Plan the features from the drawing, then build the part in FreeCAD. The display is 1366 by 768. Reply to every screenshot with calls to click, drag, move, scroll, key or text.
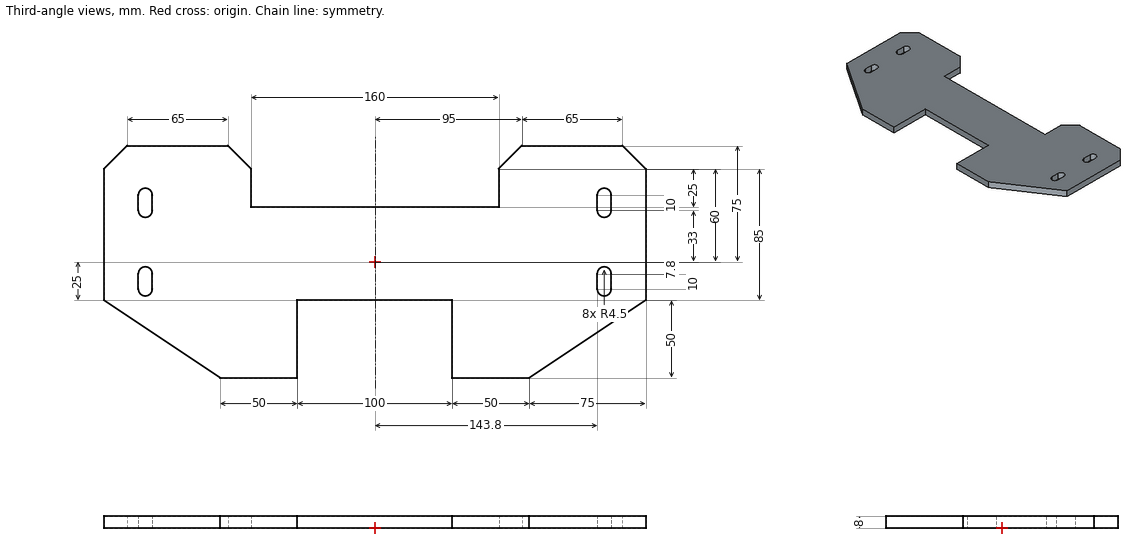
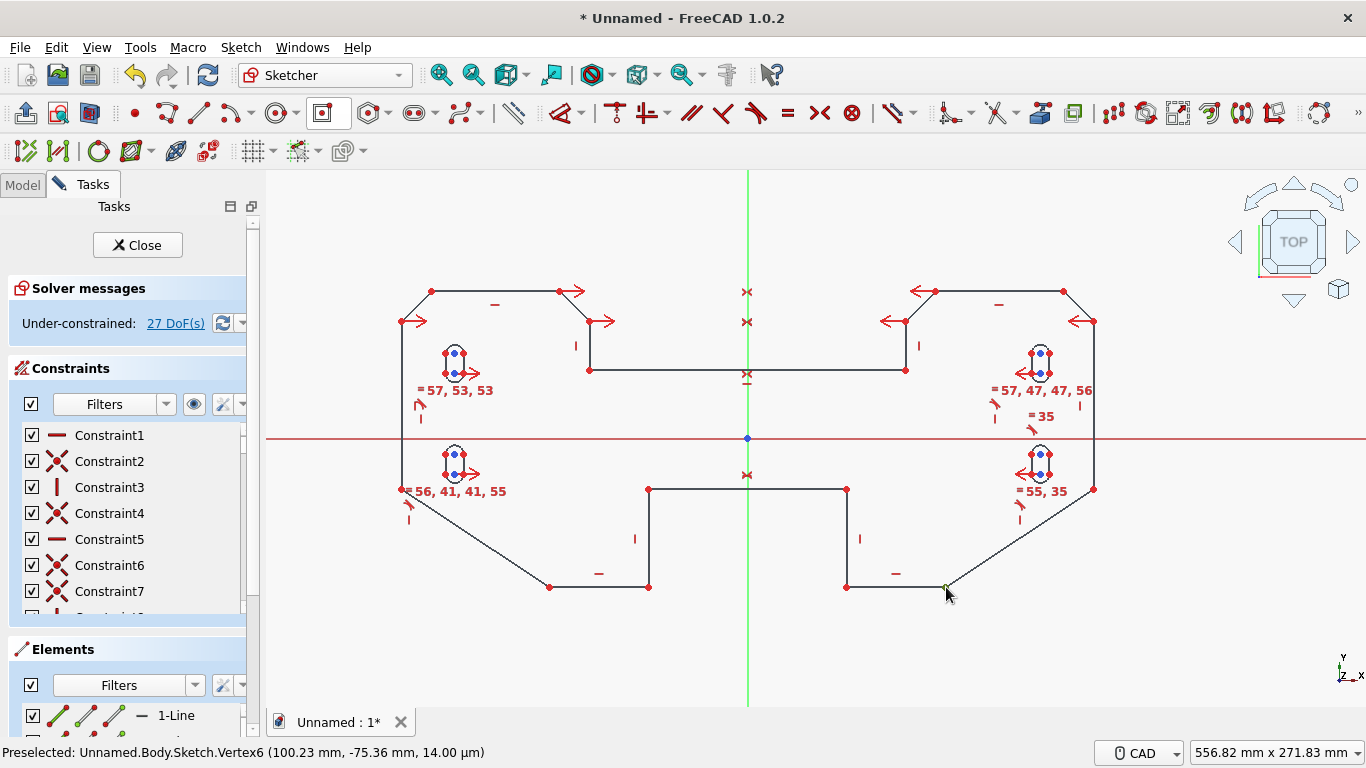
click(550, 587)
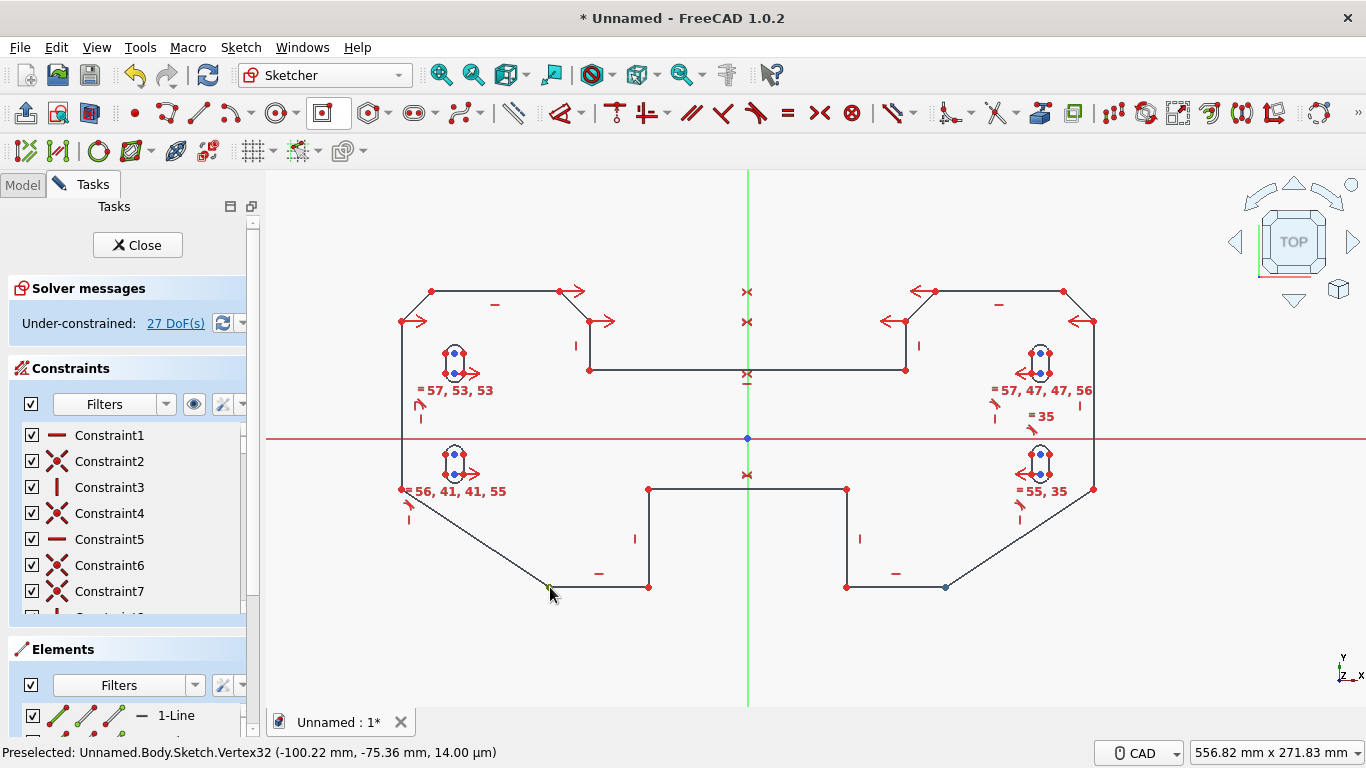
click(748, 645)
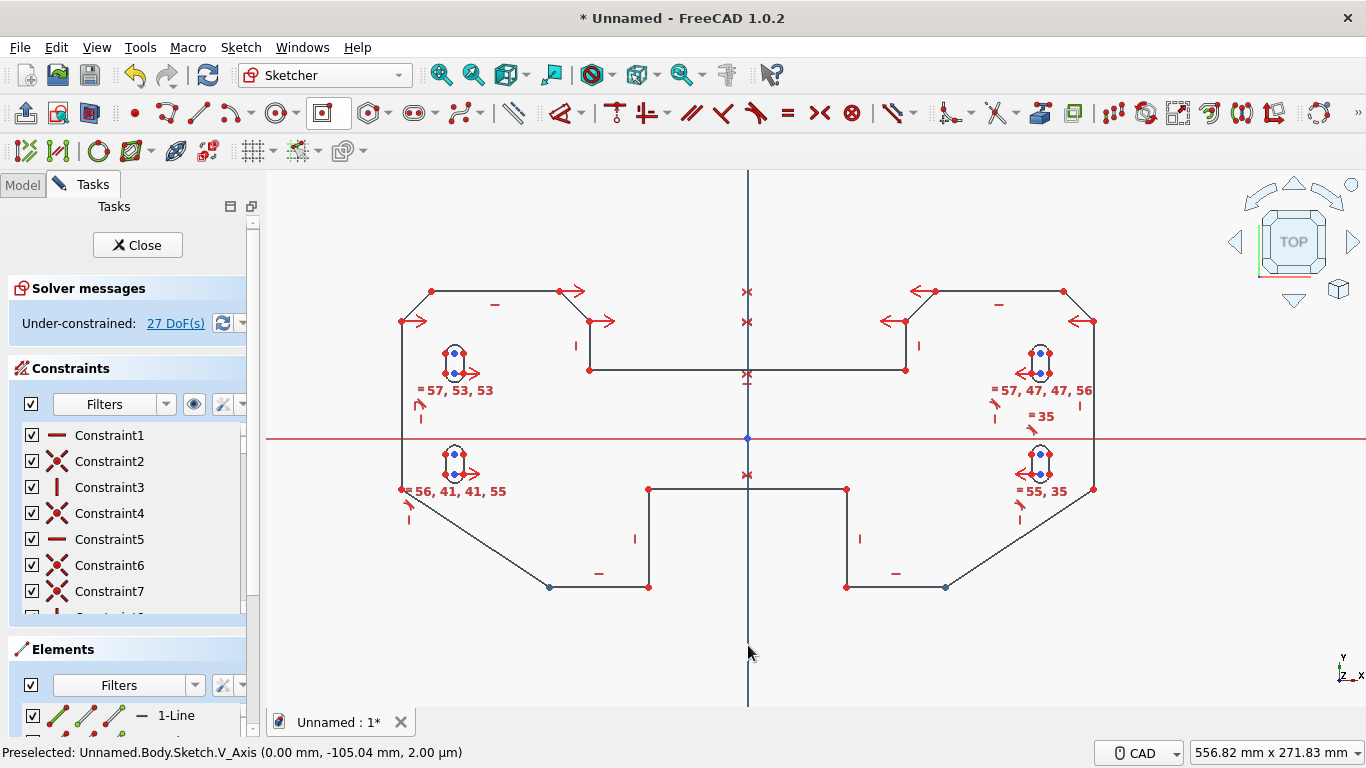
click(820, 114)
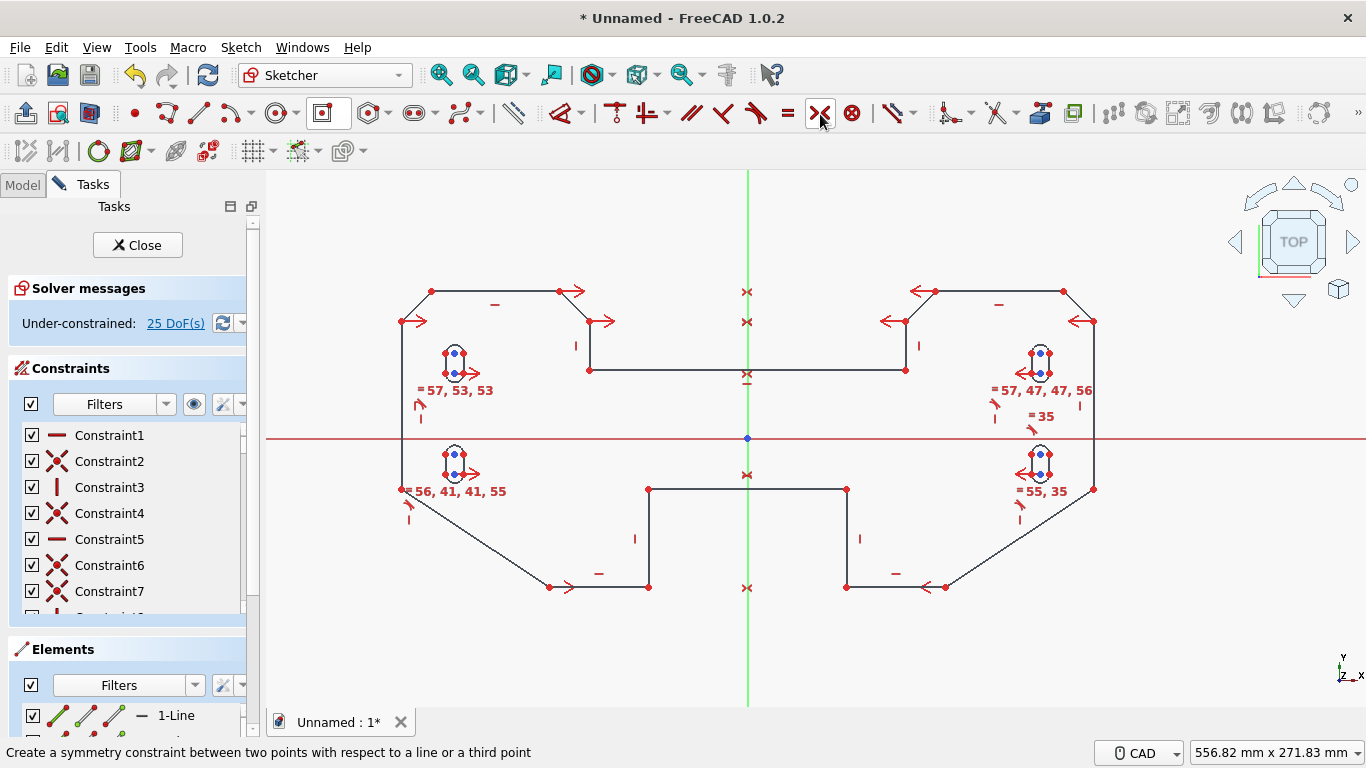
click(560, 114)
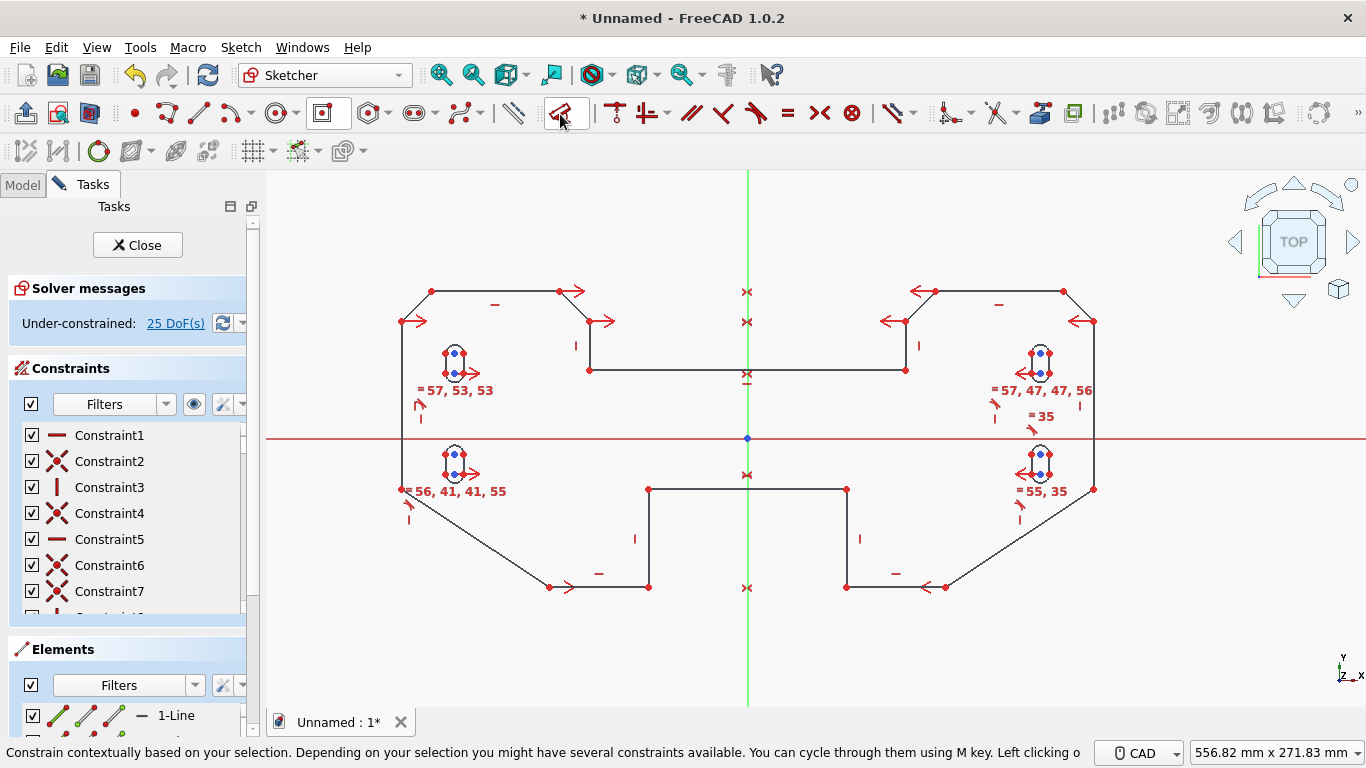
scroll(1041, 483, up, 8)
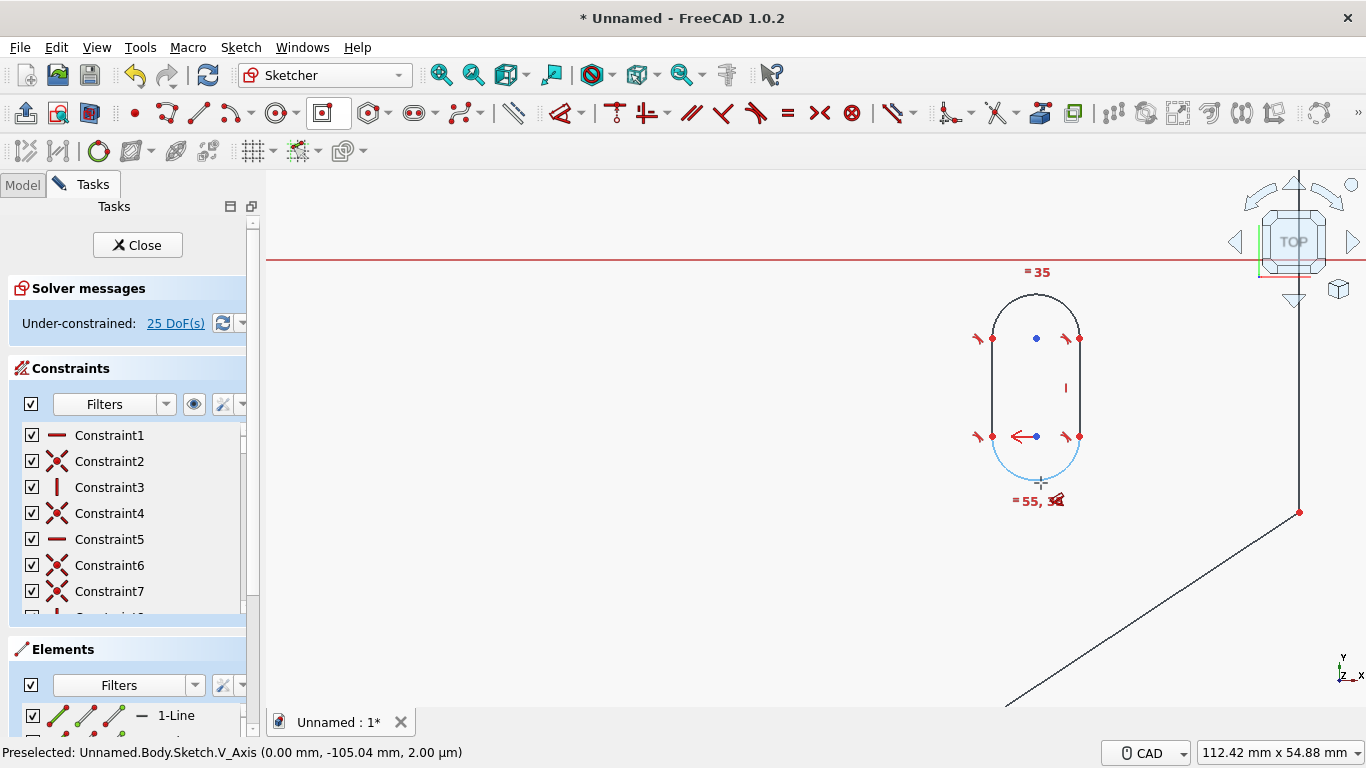
click(1036, 480)
click(1036, 512)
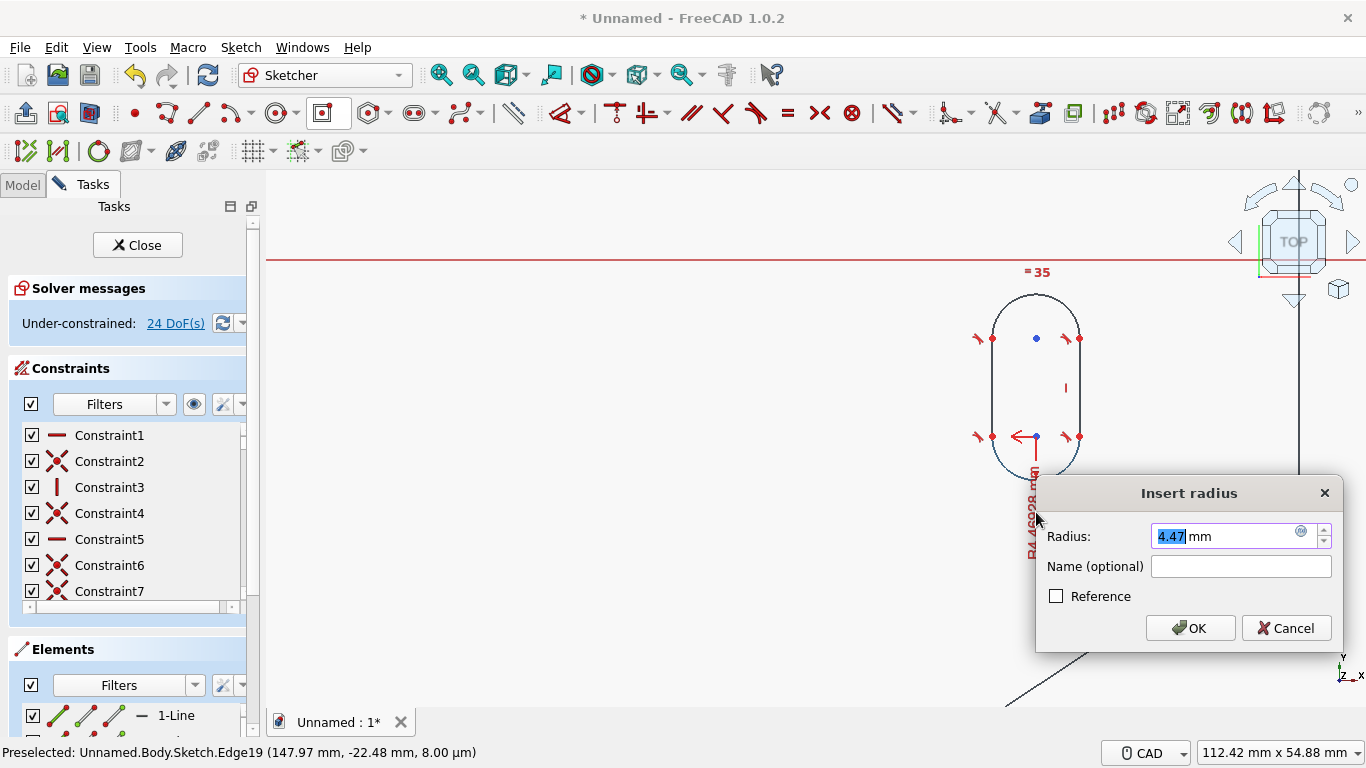
text(4.5)
key(Return)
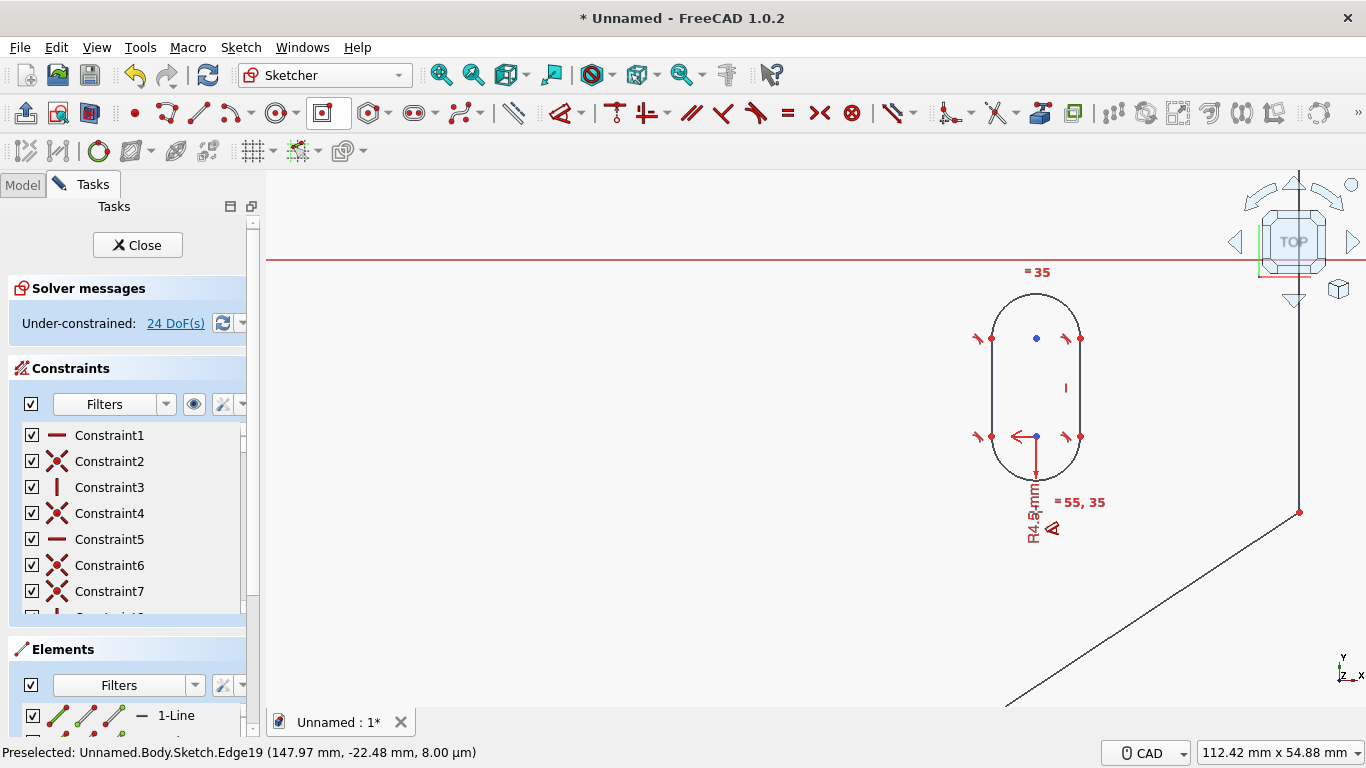
scroll(1041, 484, down, 8)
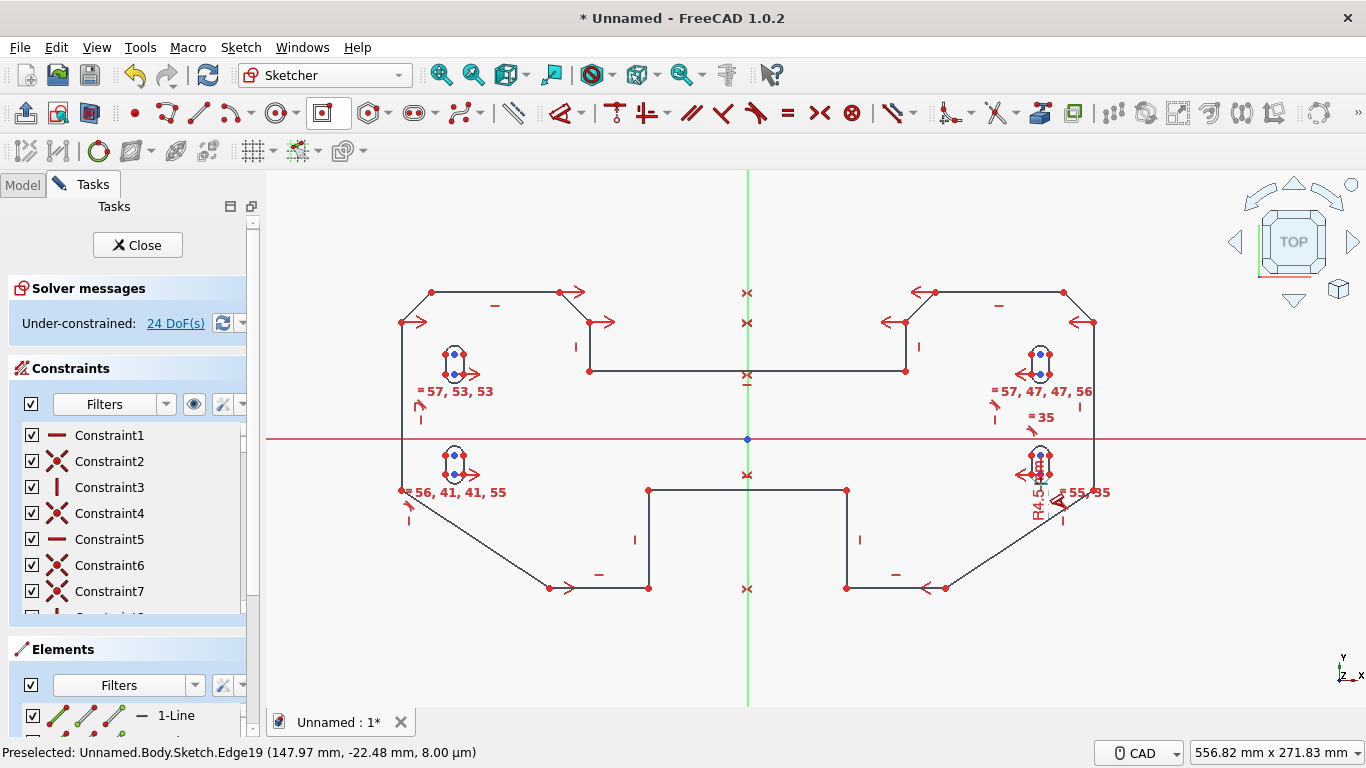
click(847, 520)
click(881, 539)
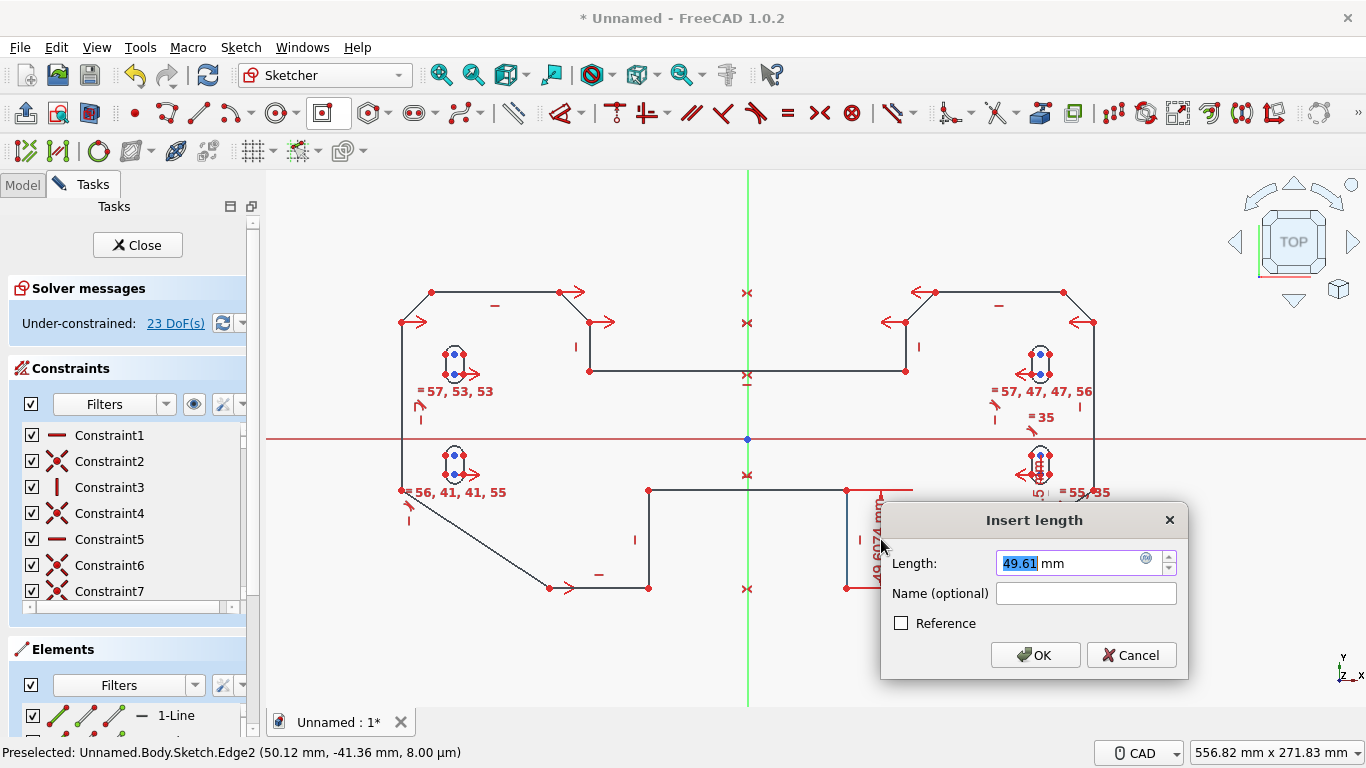
text(50)
key(Return)